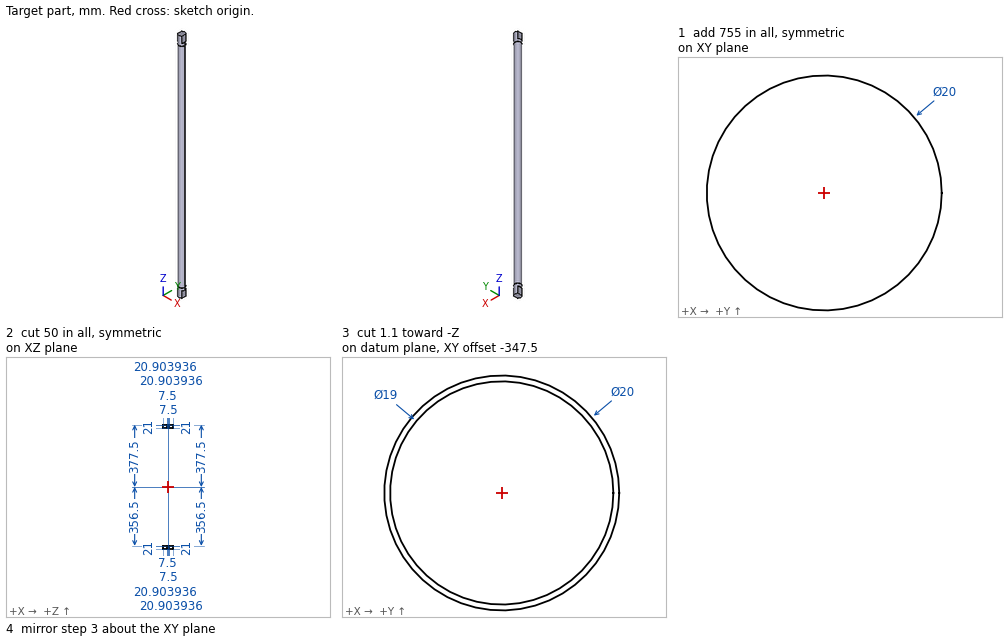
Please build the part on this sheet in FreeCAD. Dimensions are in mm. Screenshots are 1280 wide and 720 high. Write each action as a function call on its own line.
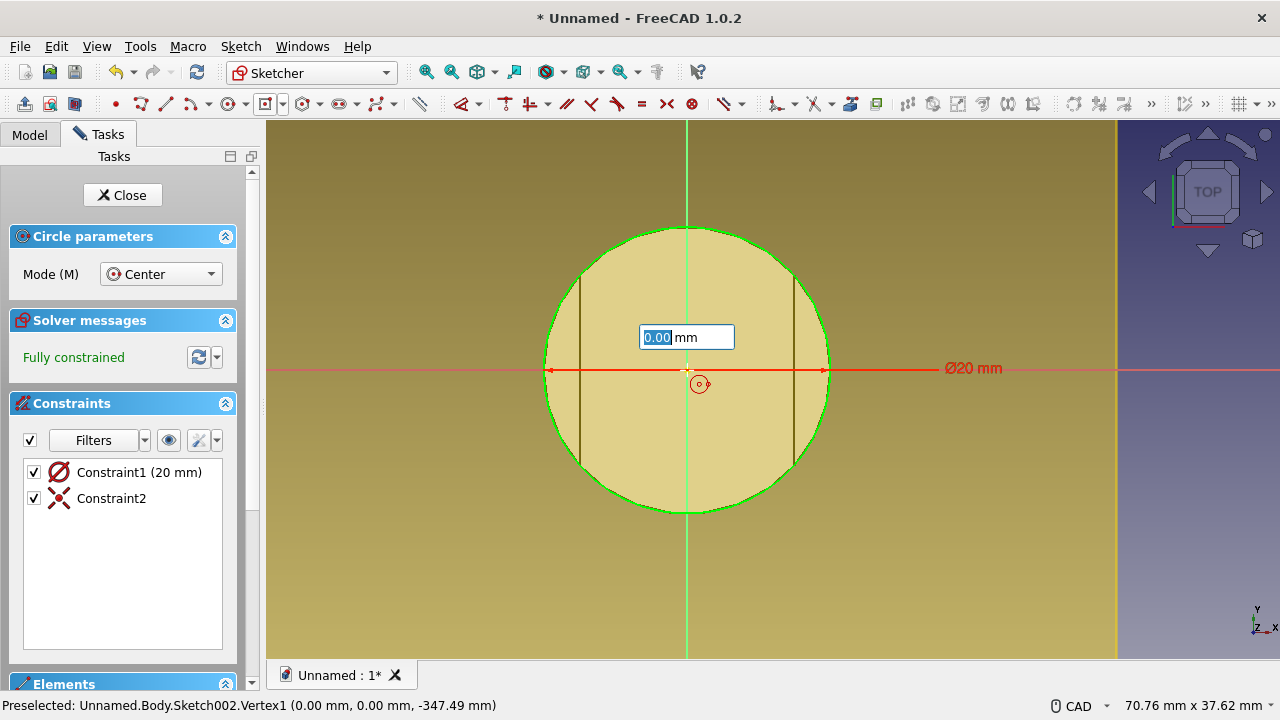
scroll(783, 274, up, 4)
move(783, 274)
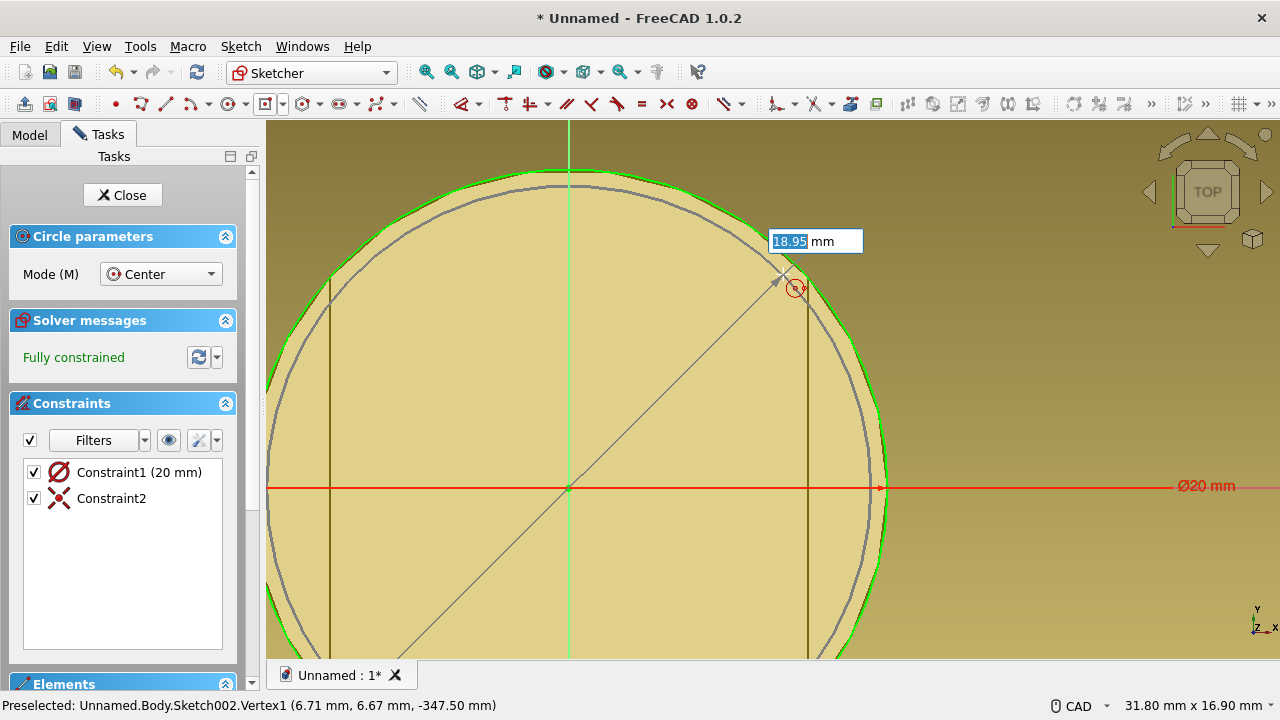
text(19)
key(Return)
key(Escape)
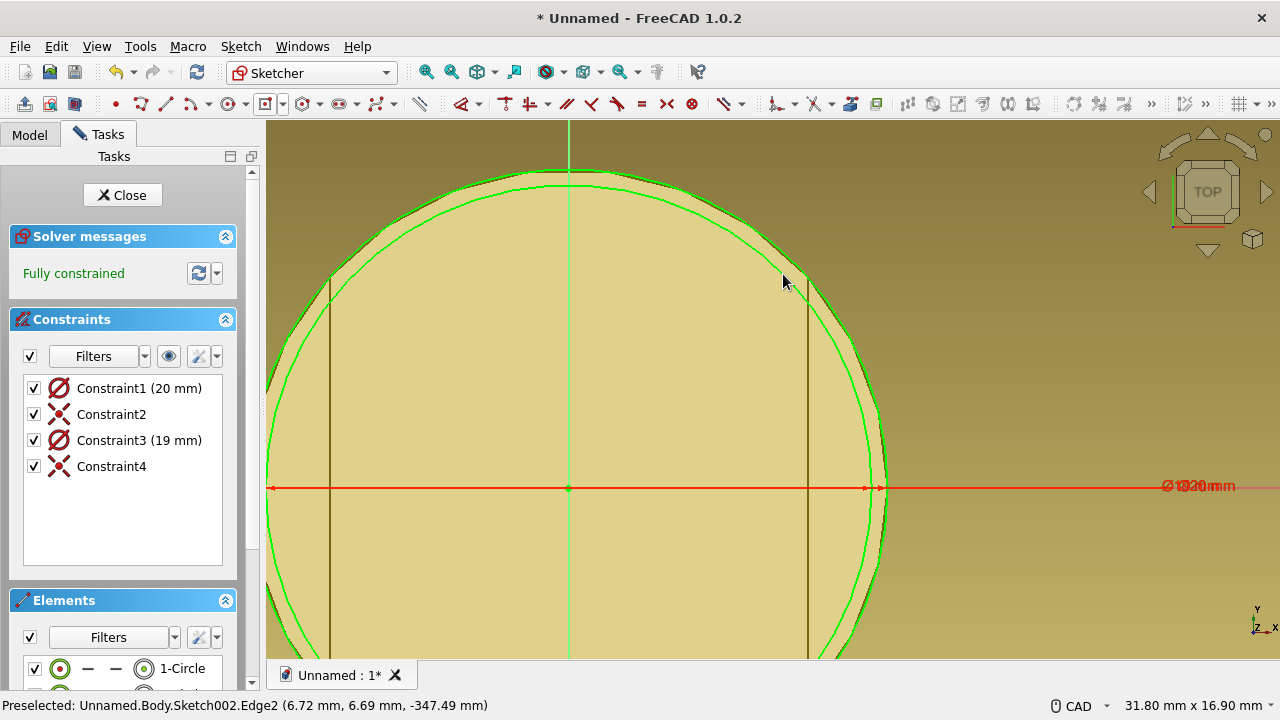
click(123, 195)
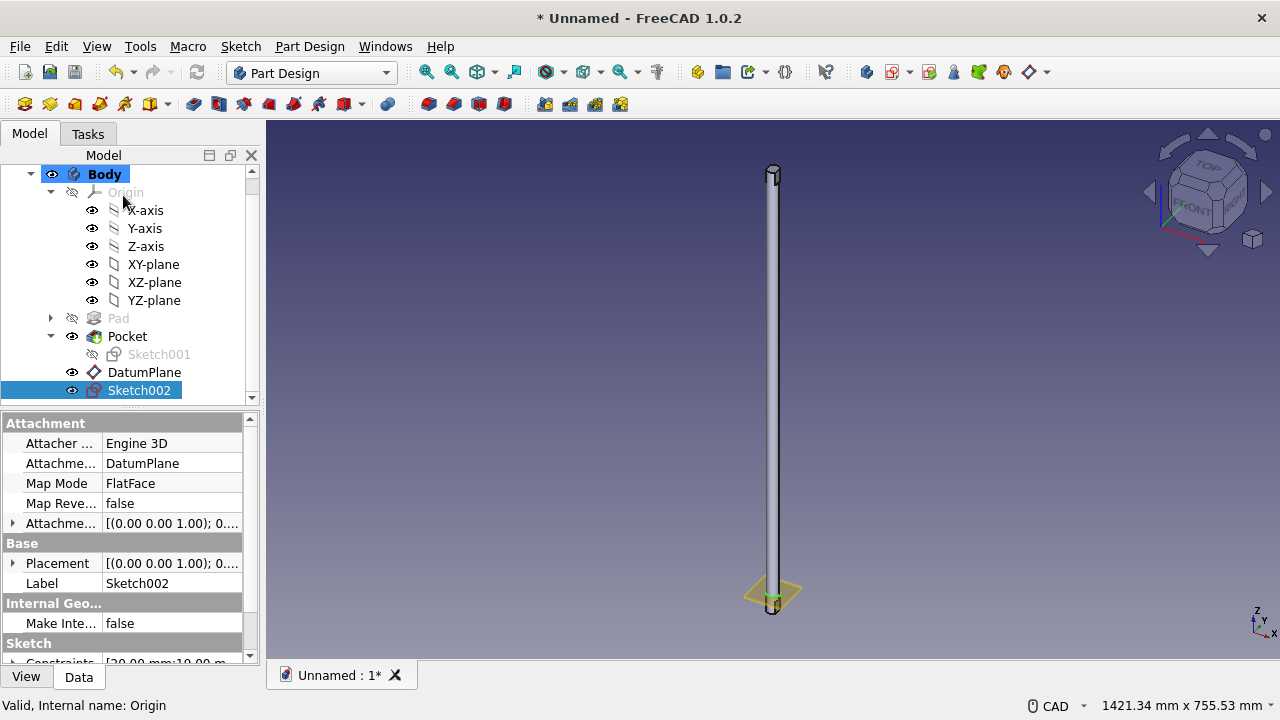
click(194, 104)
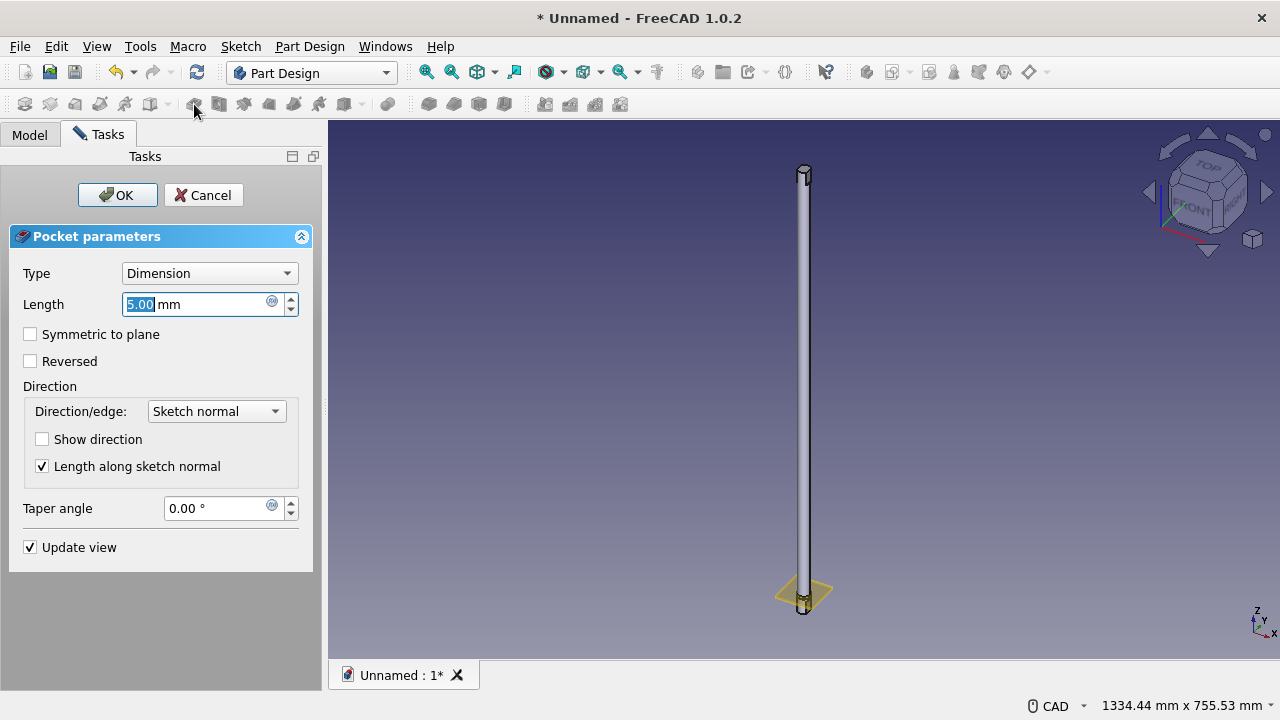
text(1.1)
key(Tab)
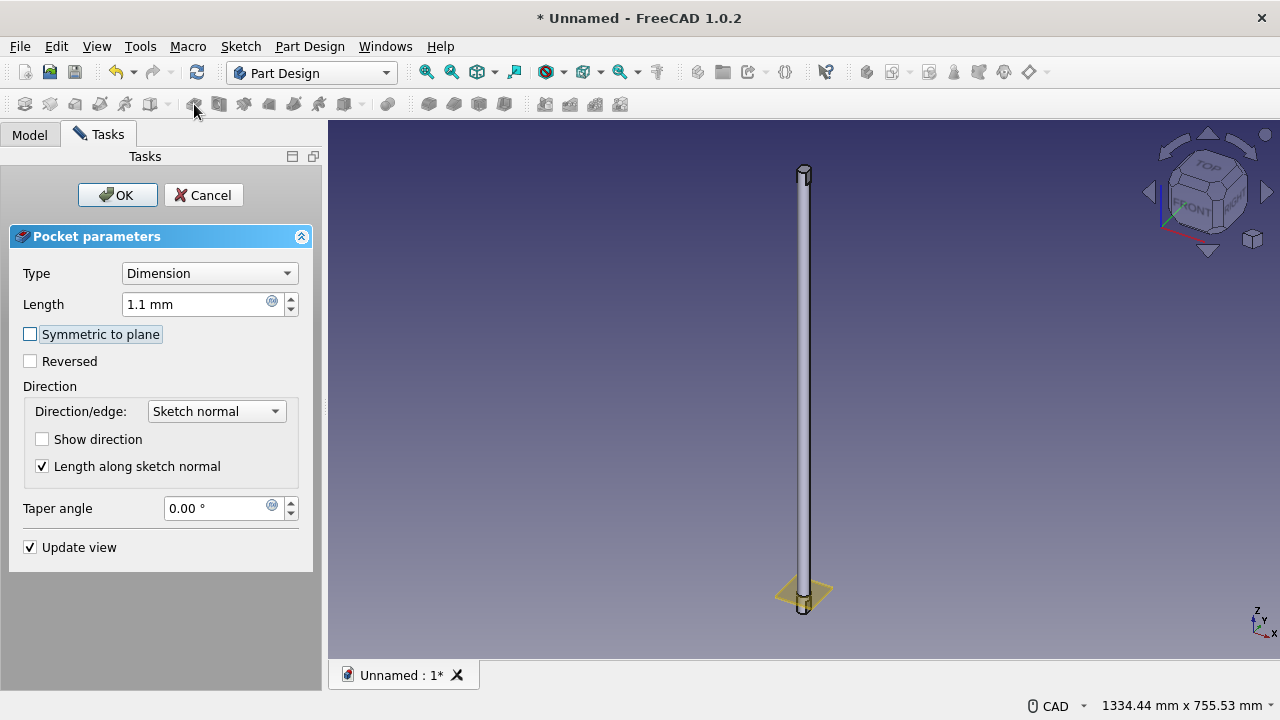
click(118, 195)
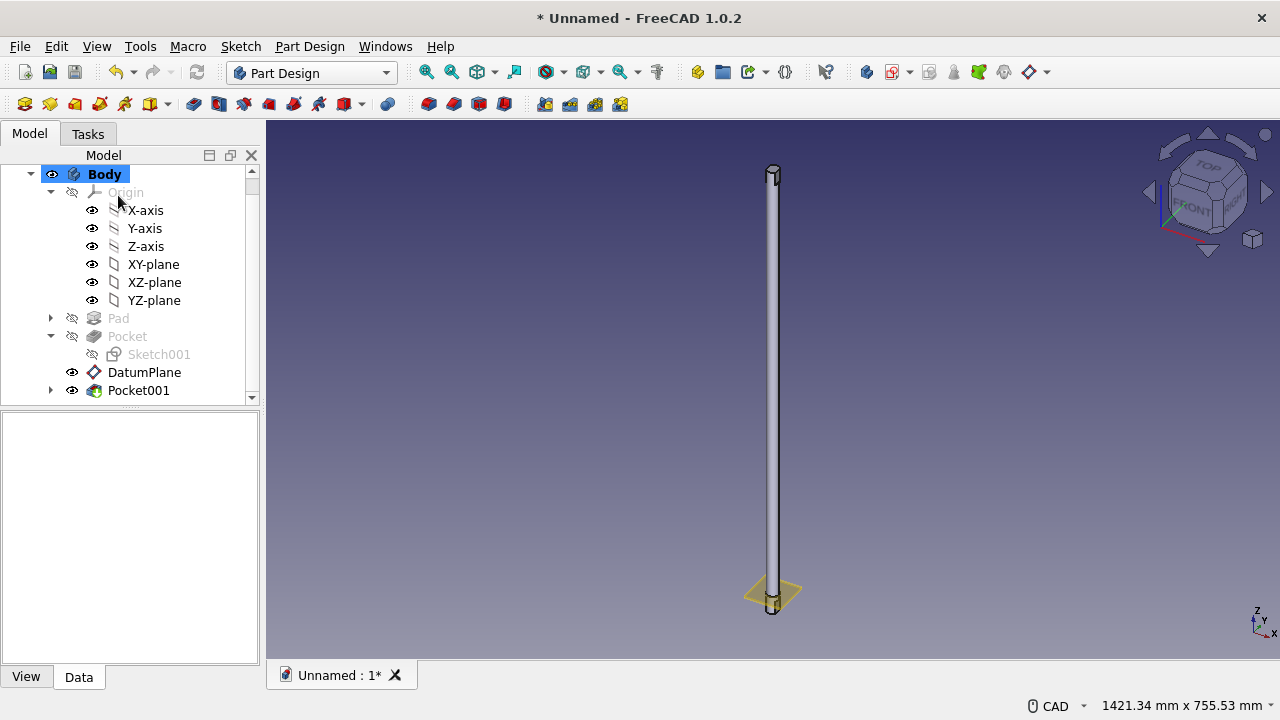
click(117, 372)
key(space)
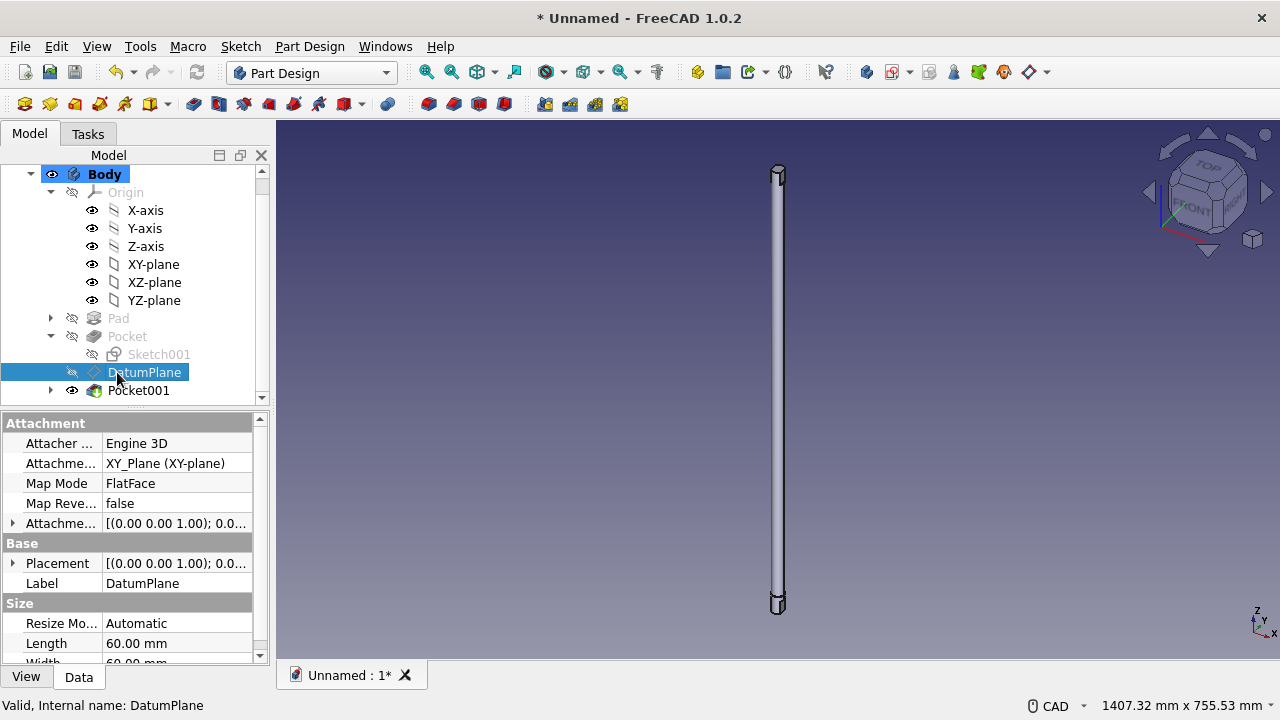
click(117, 390)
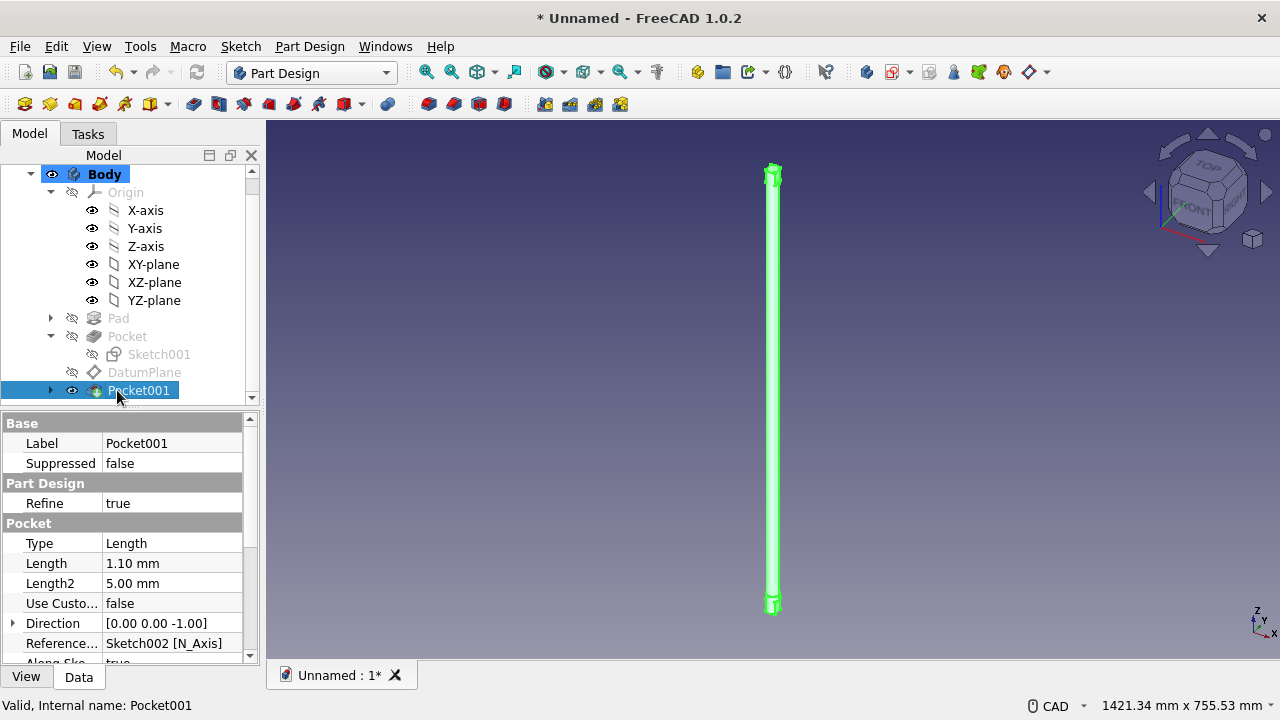
click(545, 104)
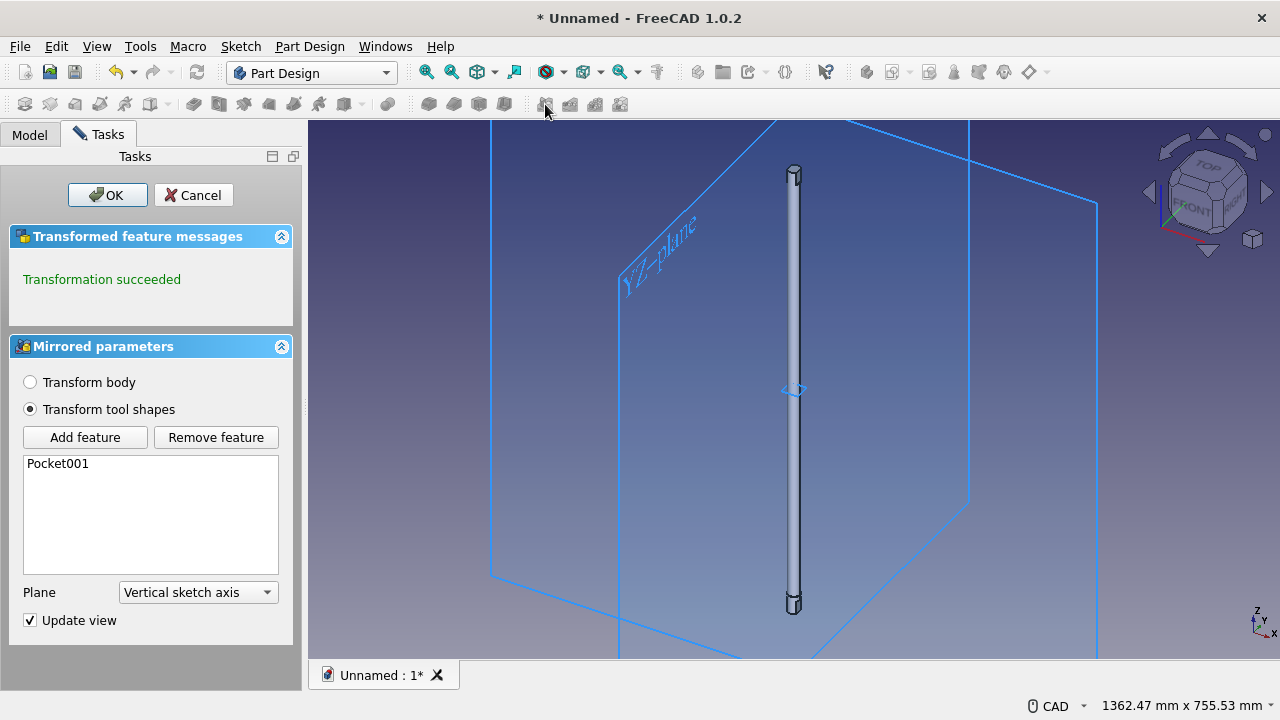
click(199, 592)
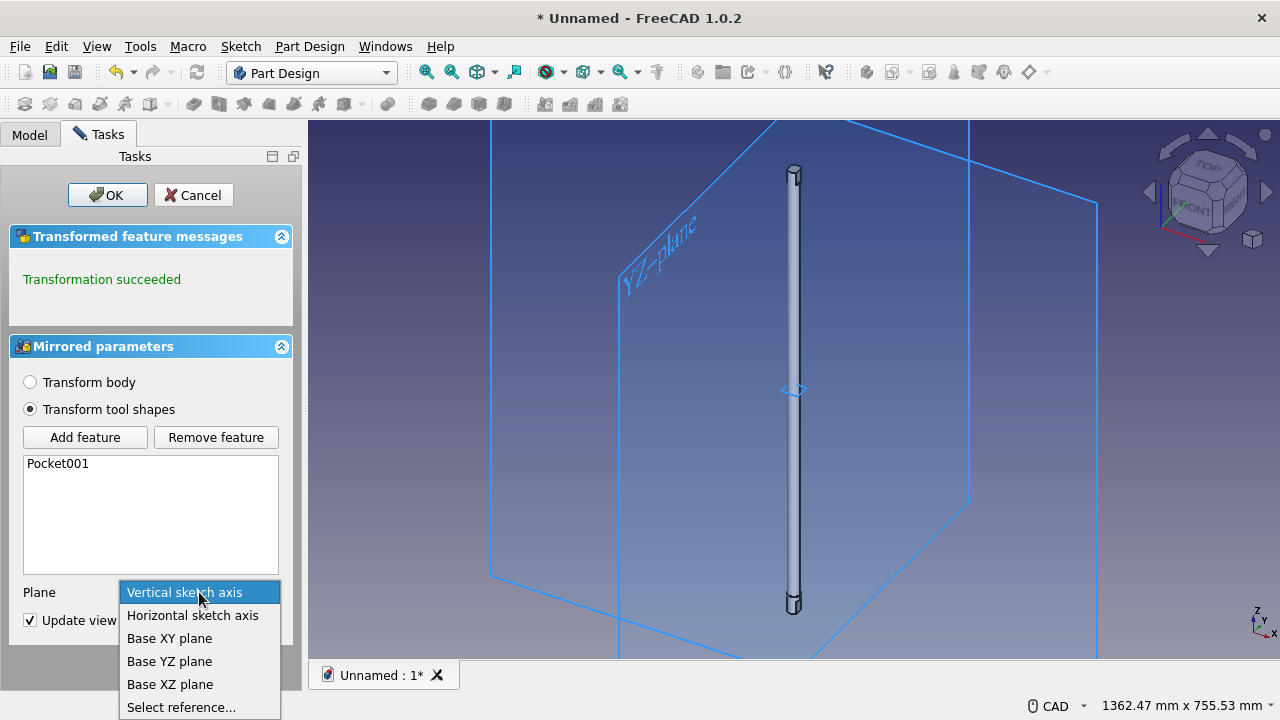
click(198, 638)